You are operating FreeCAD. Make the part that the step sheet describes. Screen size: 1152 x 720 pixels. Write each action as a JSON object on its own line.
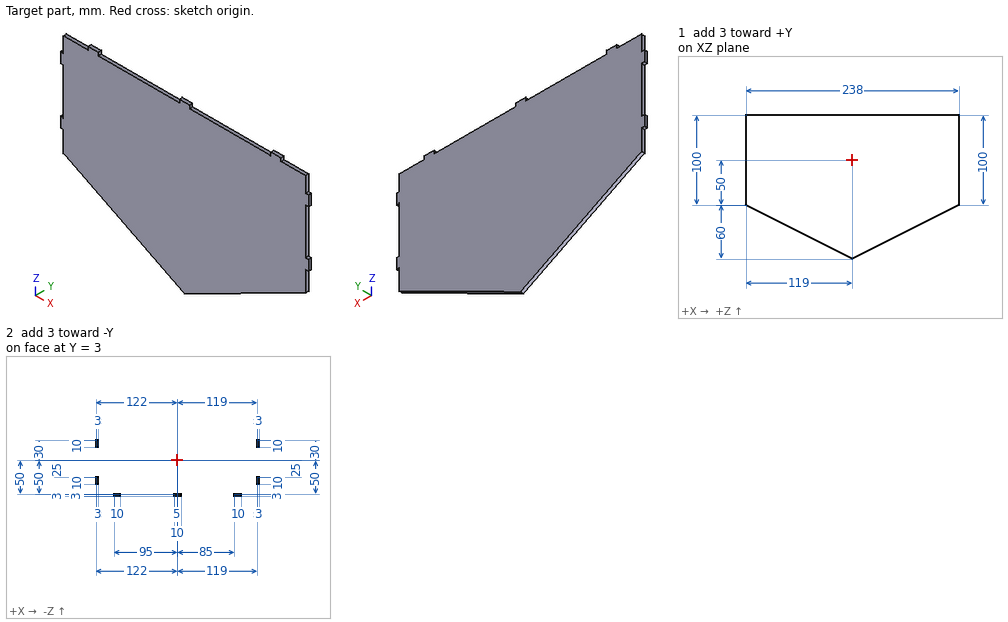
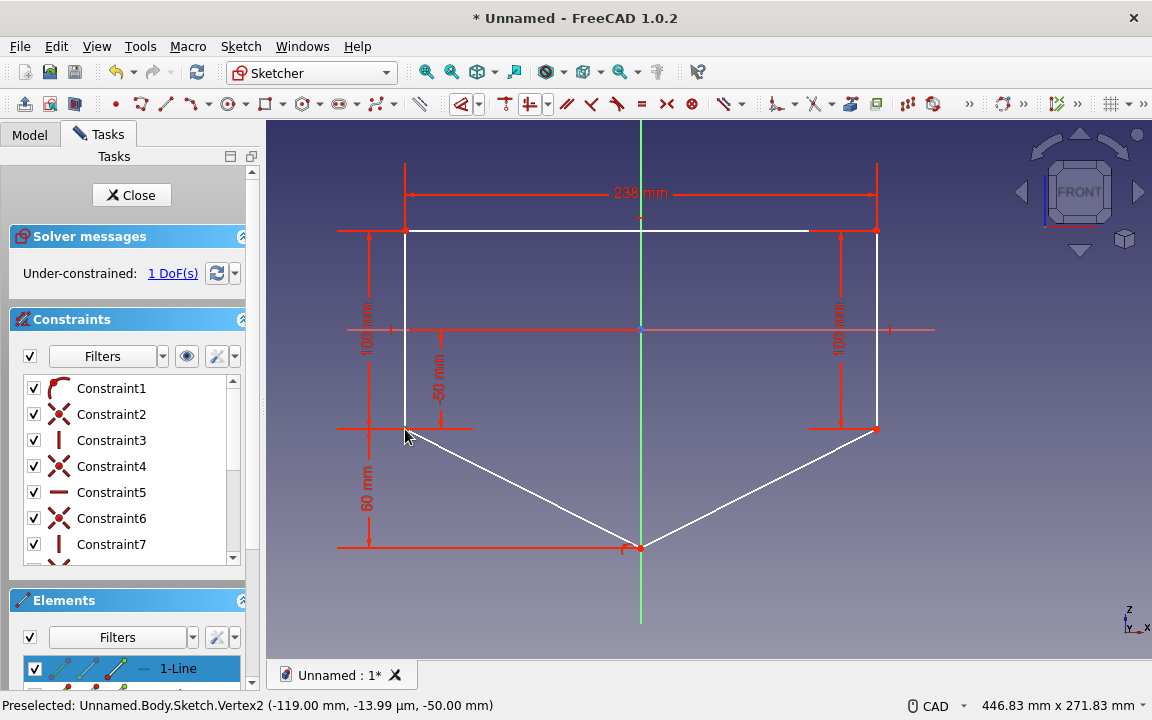
{"action": "key", "text": "l"}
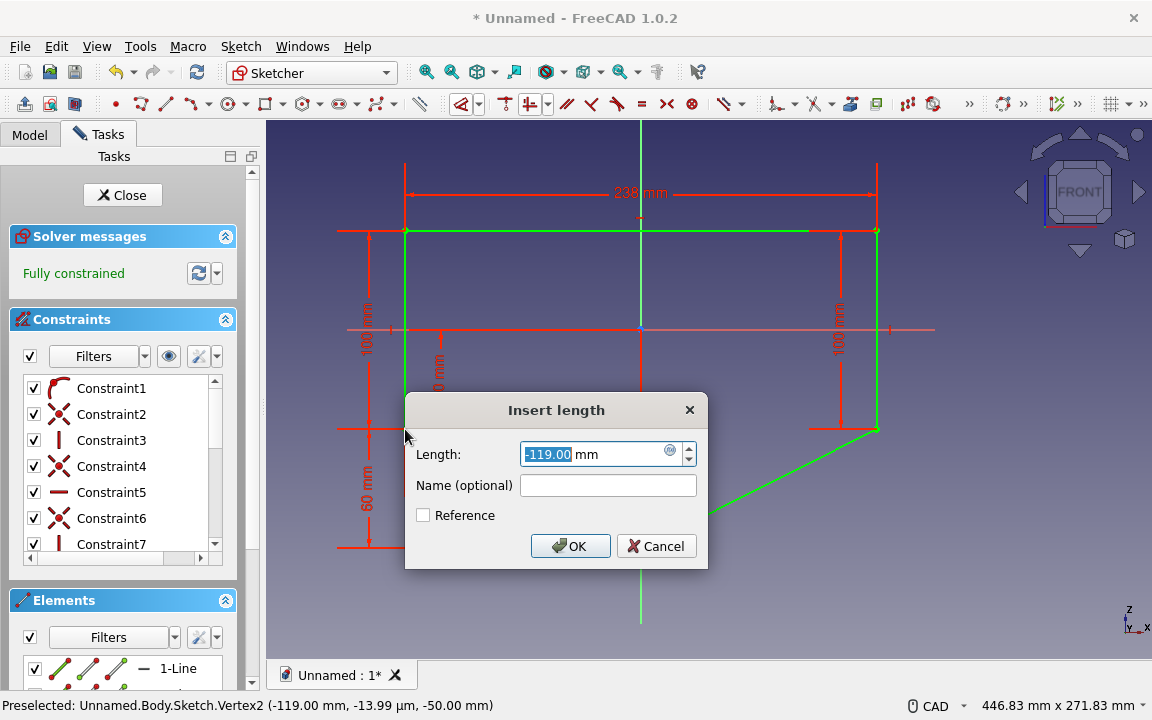
{"action": "type", "text": "-119"}
{"action": "key", "text": "Return"}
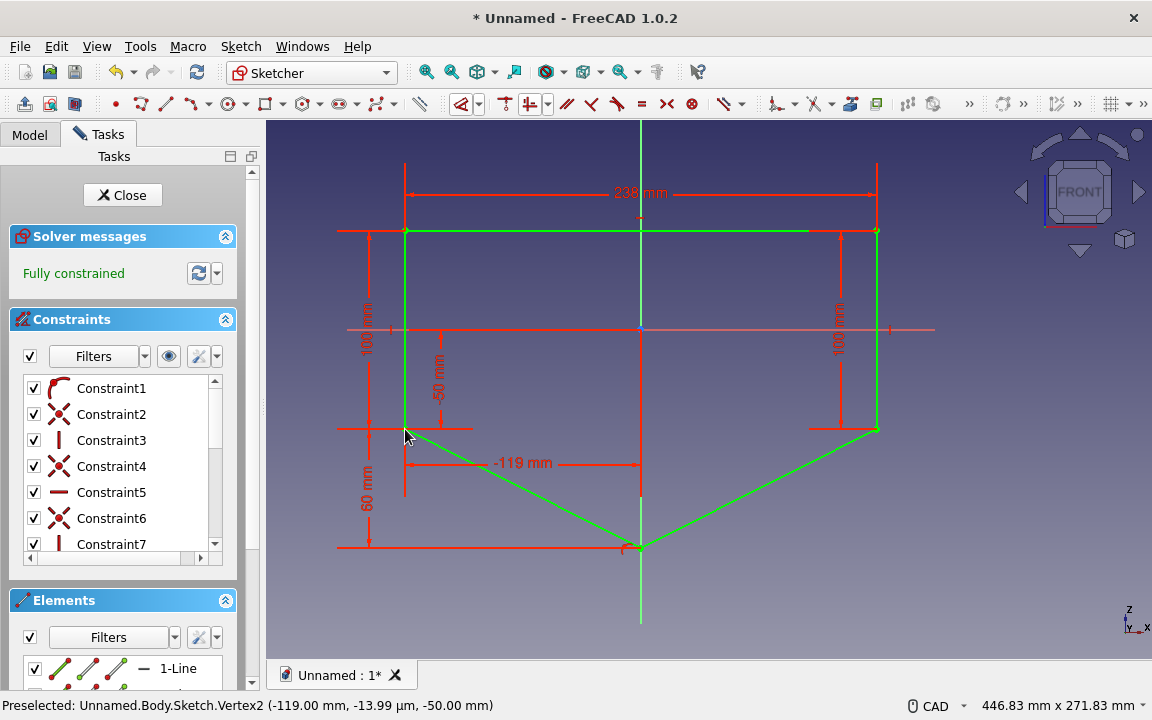
{"action": "left_click", "coordinate": [123, 195]}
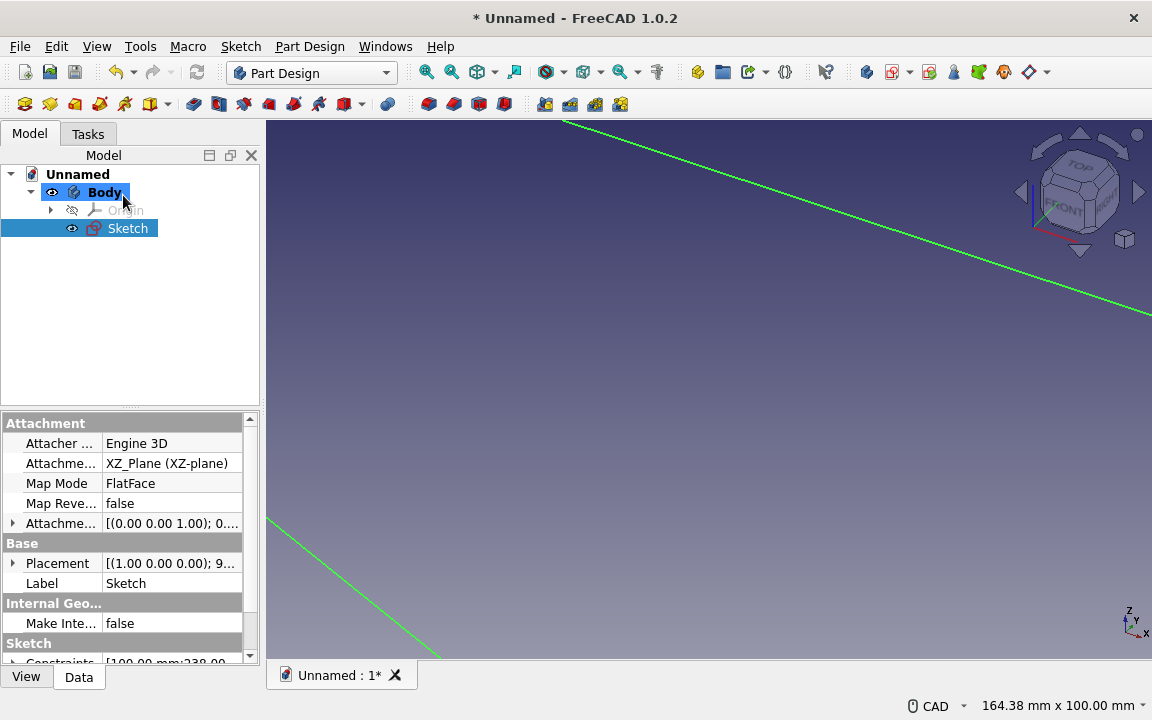
{"action": "left_click", "coordinate": [25, 104]}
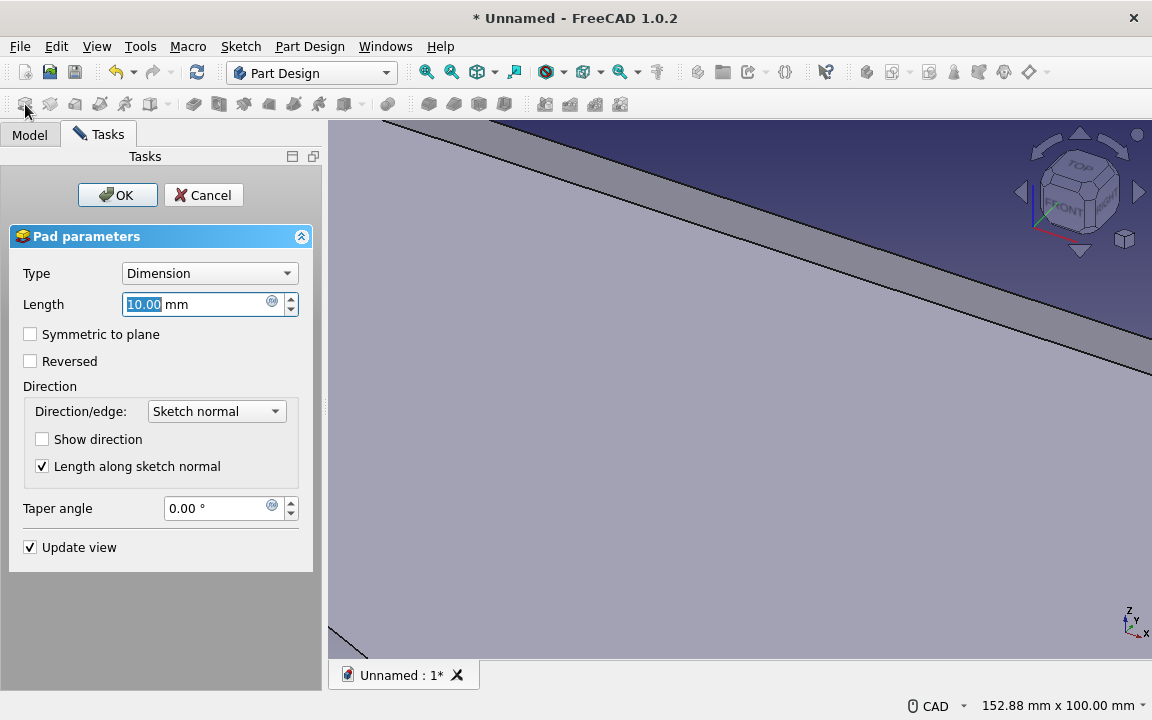
{"action": "type", "text": "3"}
{"action": "key", "text": "Tab"}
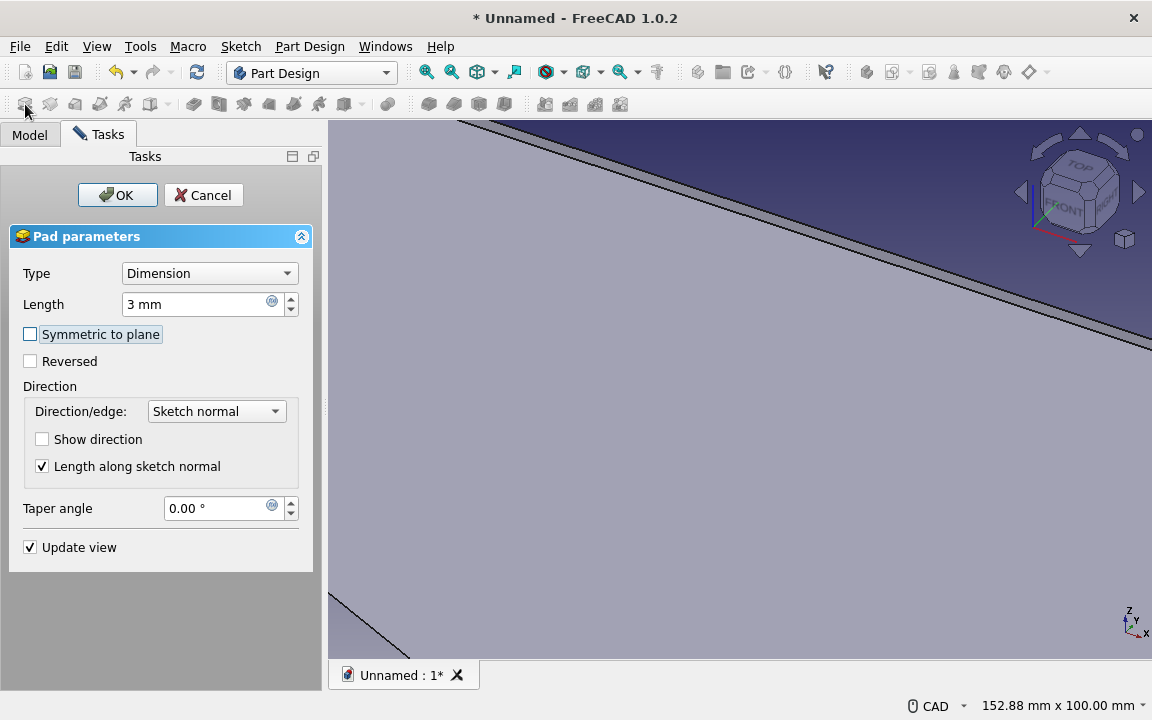
{"action": "left_click", "coordinate": [31, 361]}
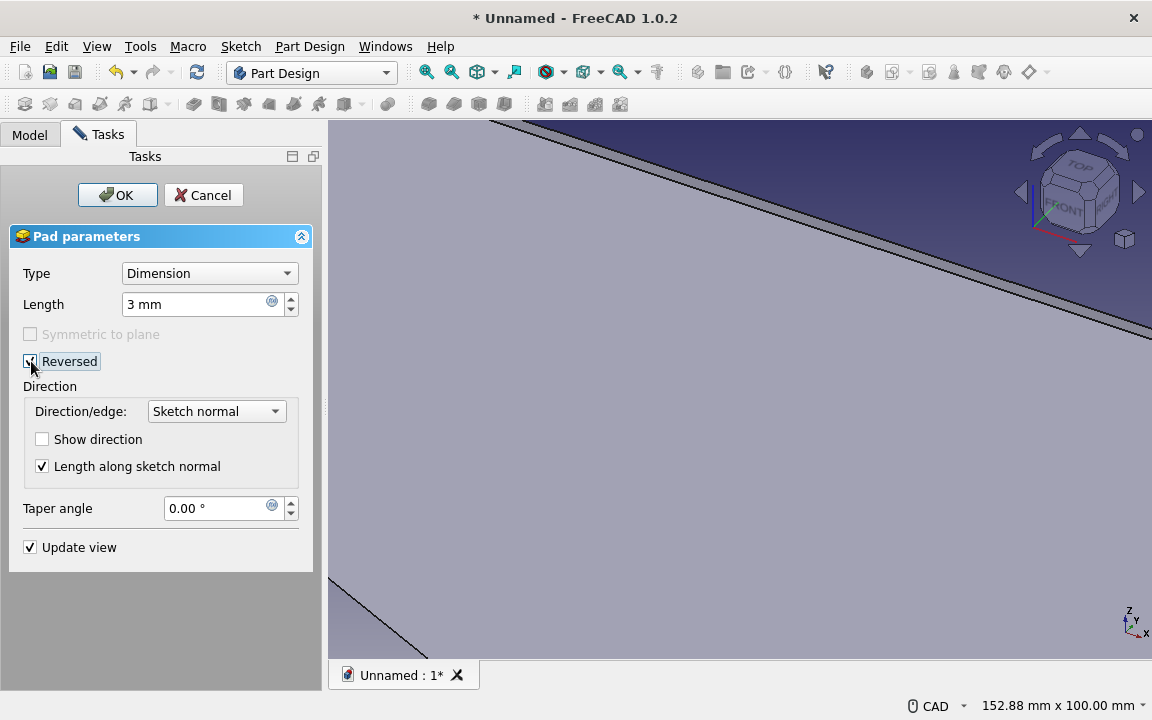
{"action": "left_click", "coordinate": [118, 195]}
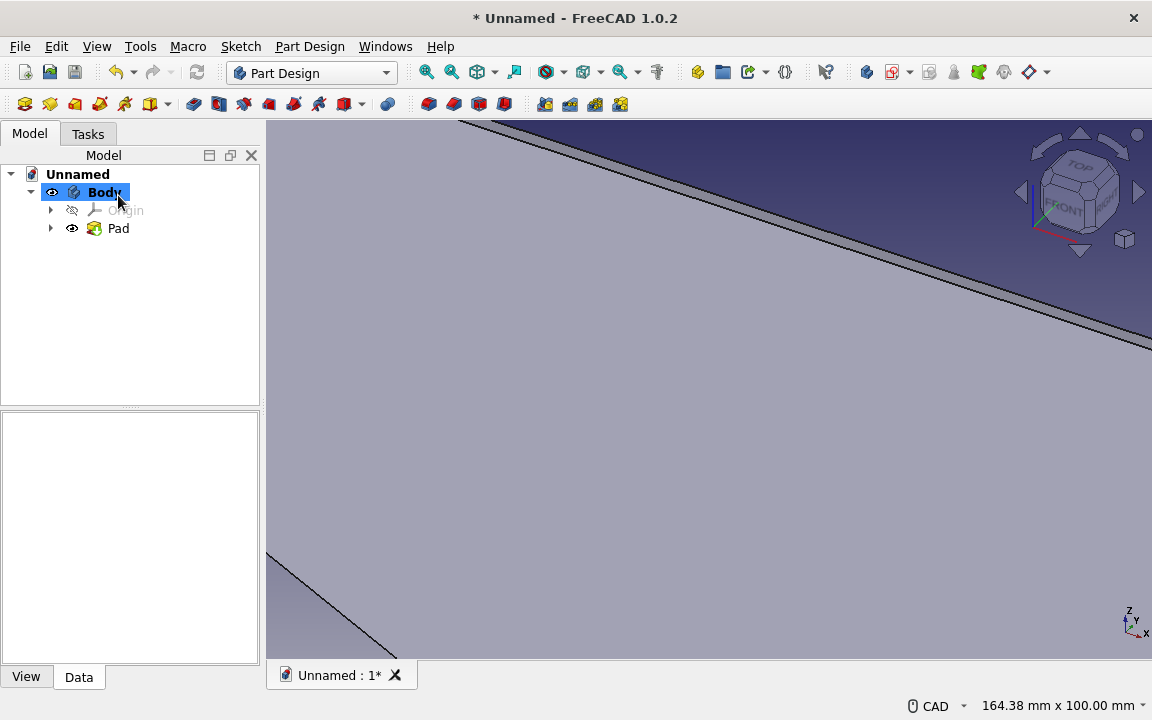
{"action": "key", "text": "v f"}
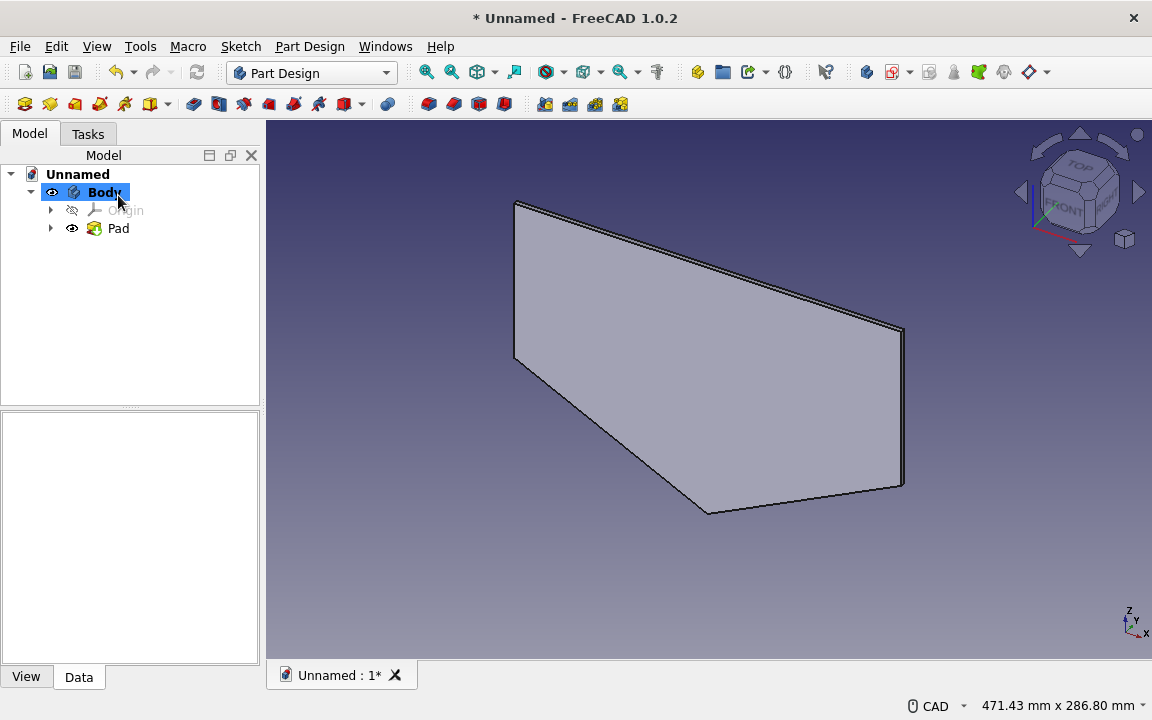
{"action": "key", "text": "4"}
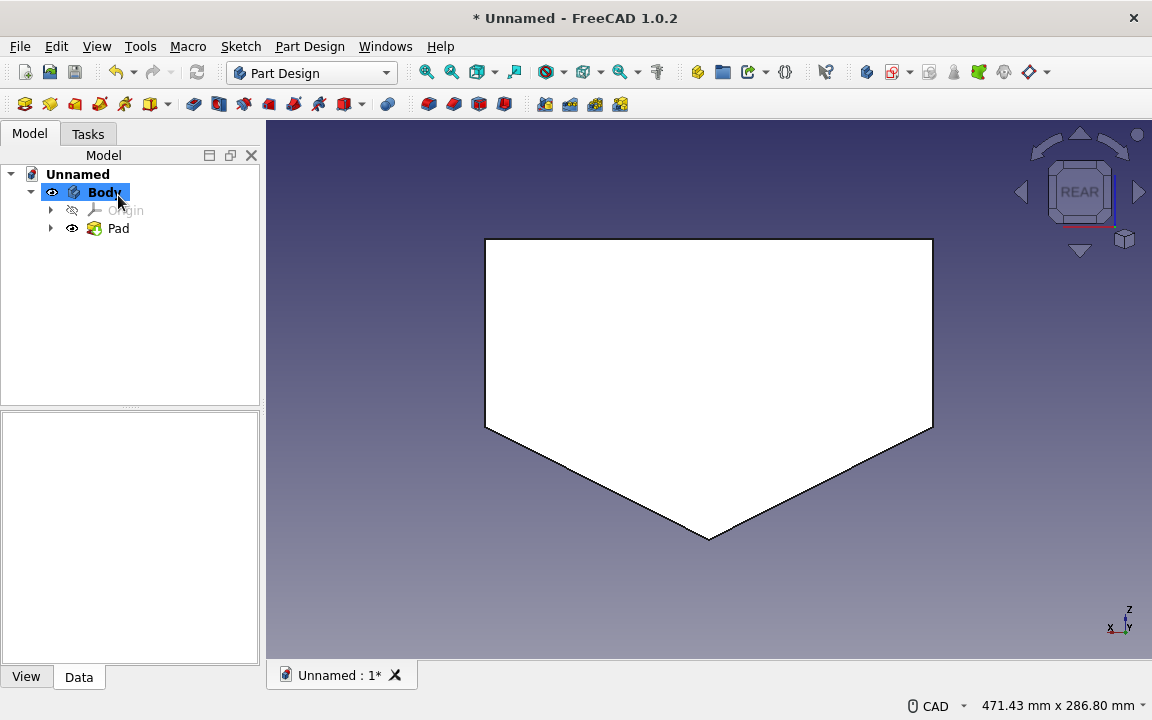
{"action": "left_click", "coordinate": [709, 388]}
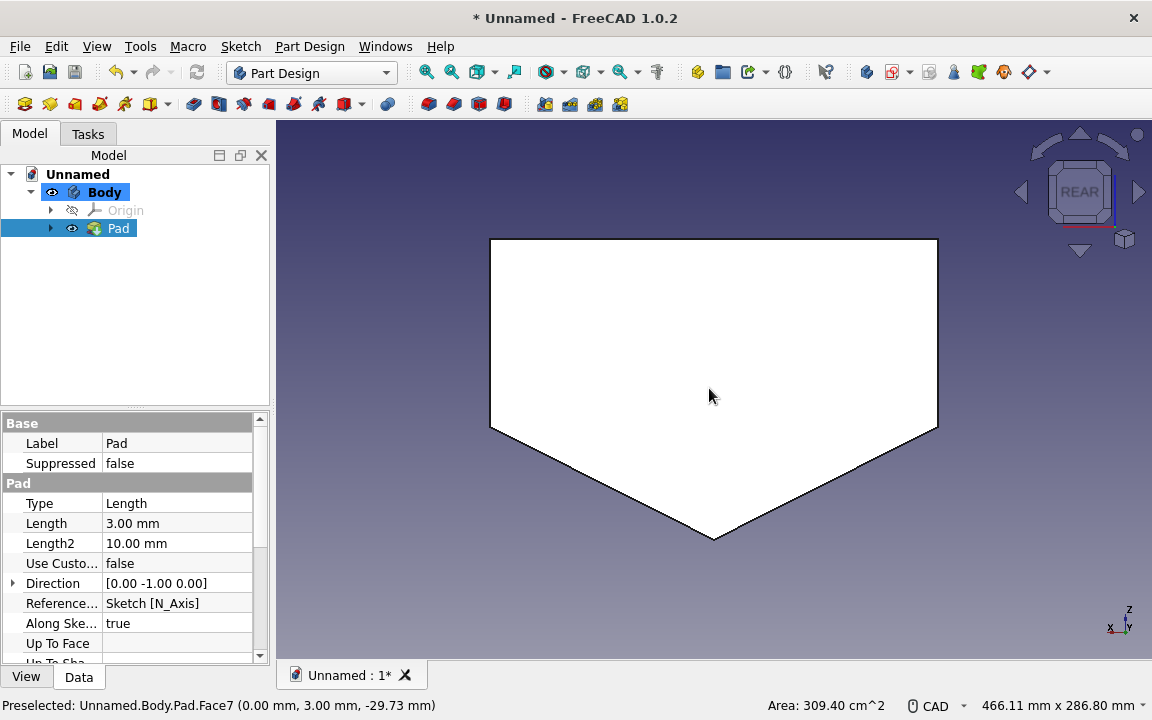
{"action": "left_click", "coordinate": [892, 72]}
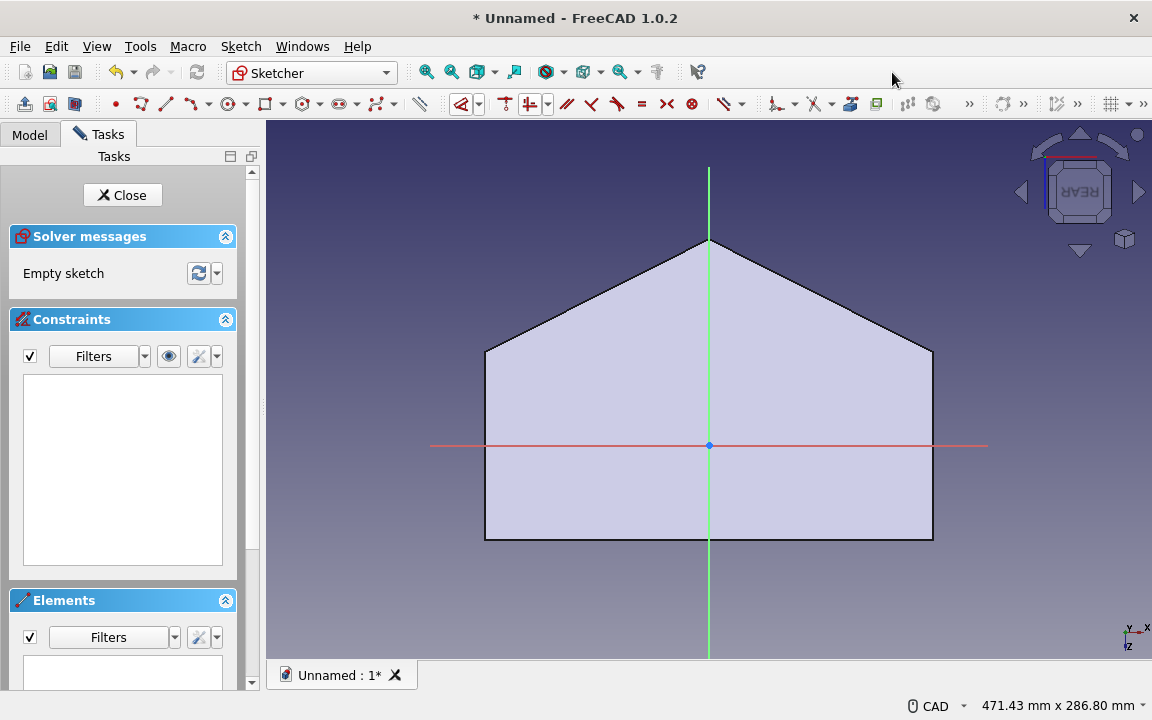
{"action": "left_click", "coordinate": [264, 104]}